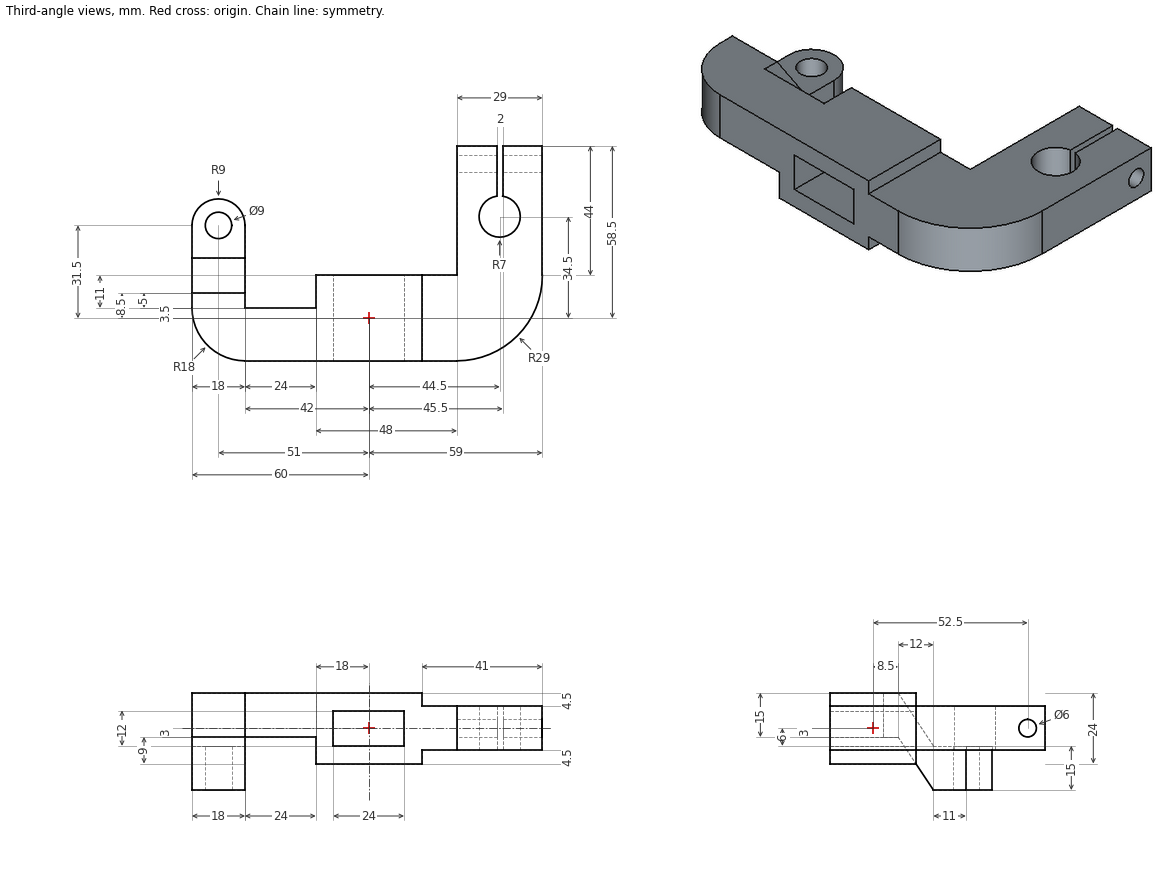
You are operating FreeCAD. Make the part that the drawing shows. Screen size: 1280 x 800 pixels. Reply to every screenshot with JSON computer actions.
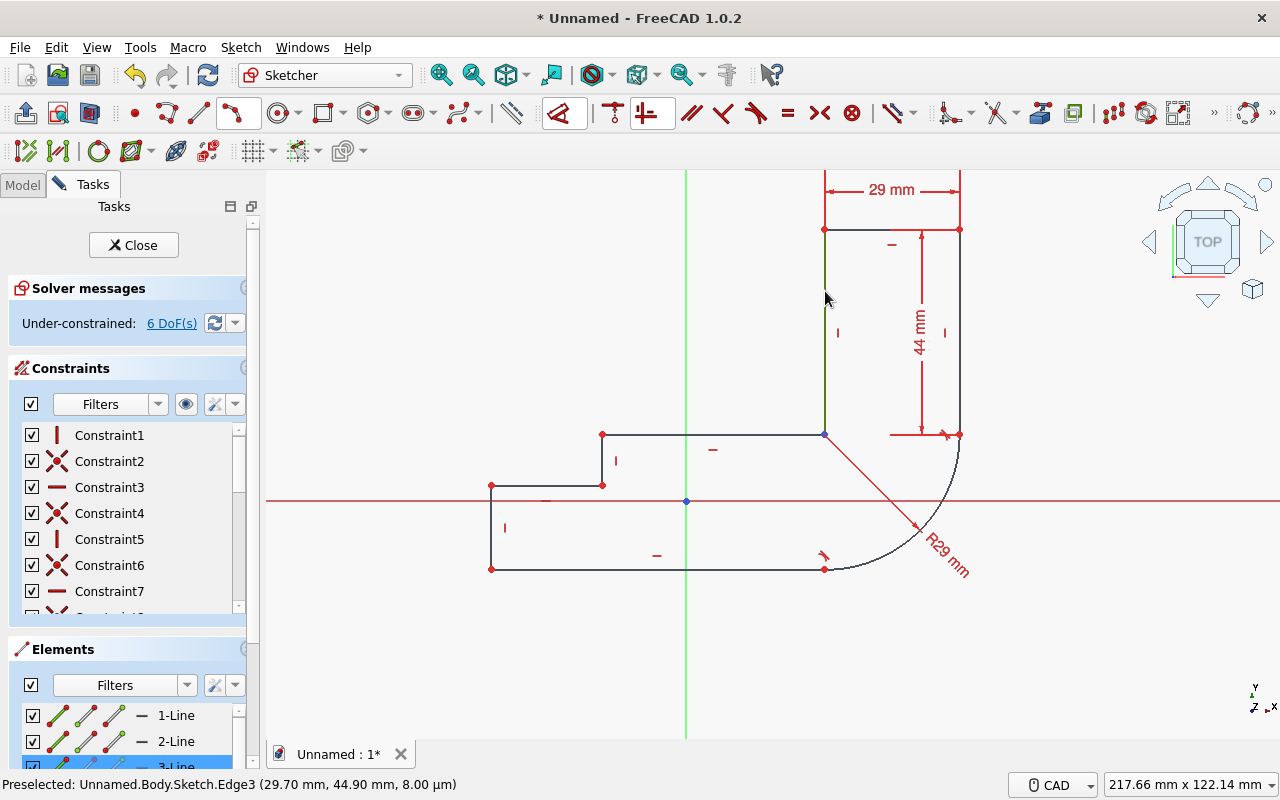
{"action": "key", "text": "i"}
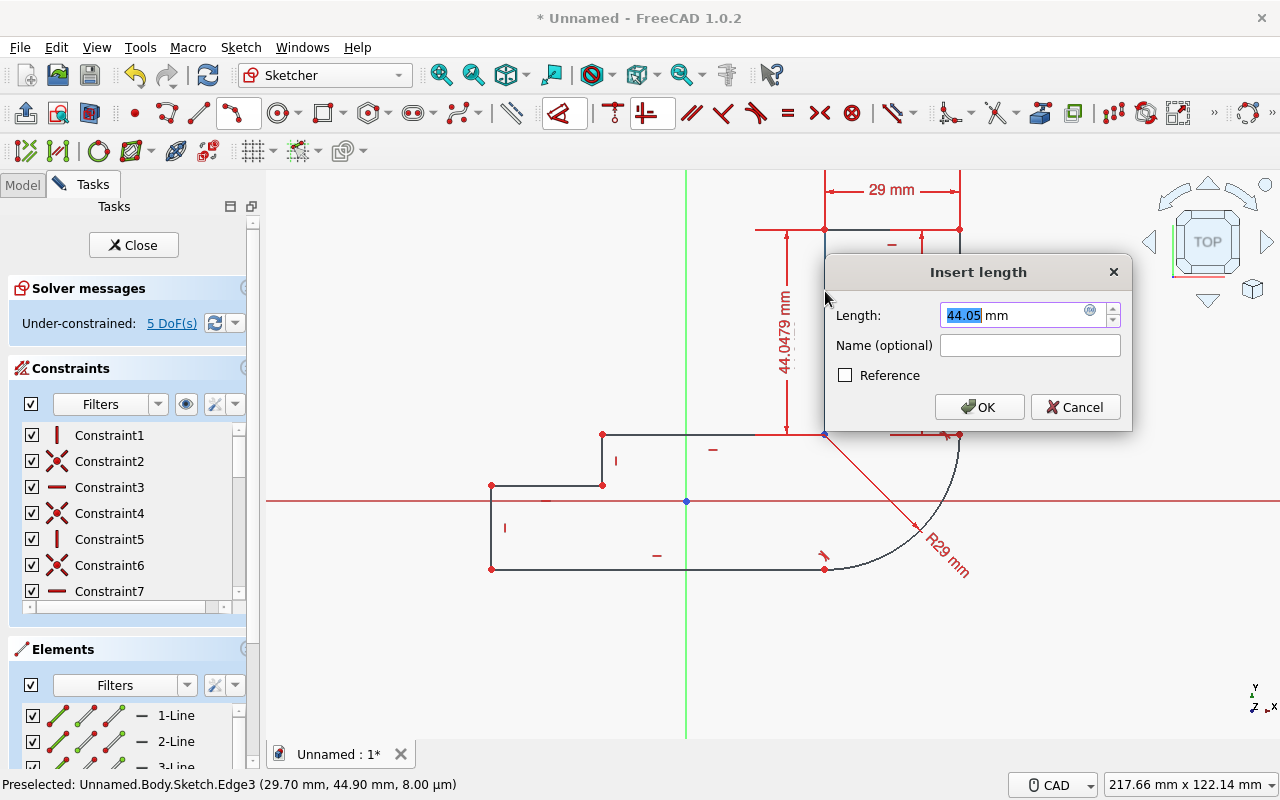
{"action": "type", "text": "44"}
{"action": "key", "text": "Return"}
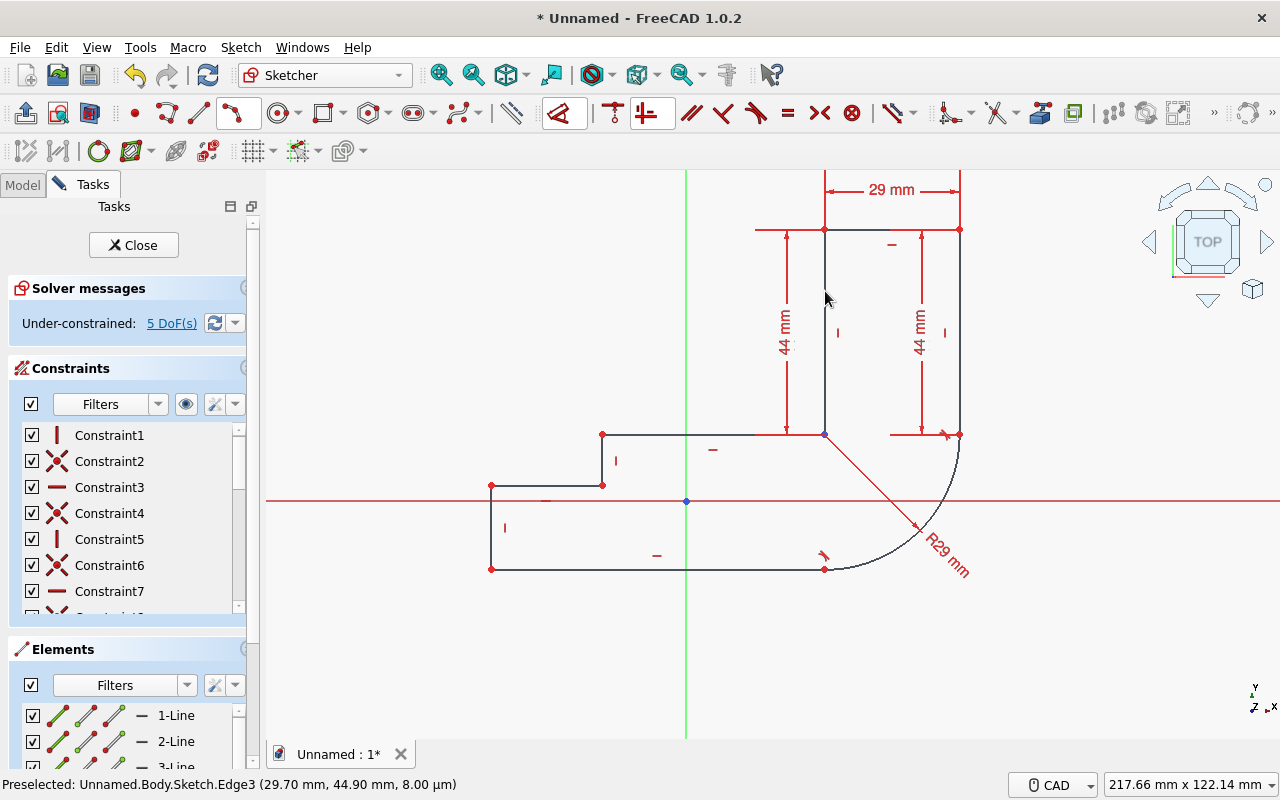
{"action": "left_click", "coordinate": [758, 435]}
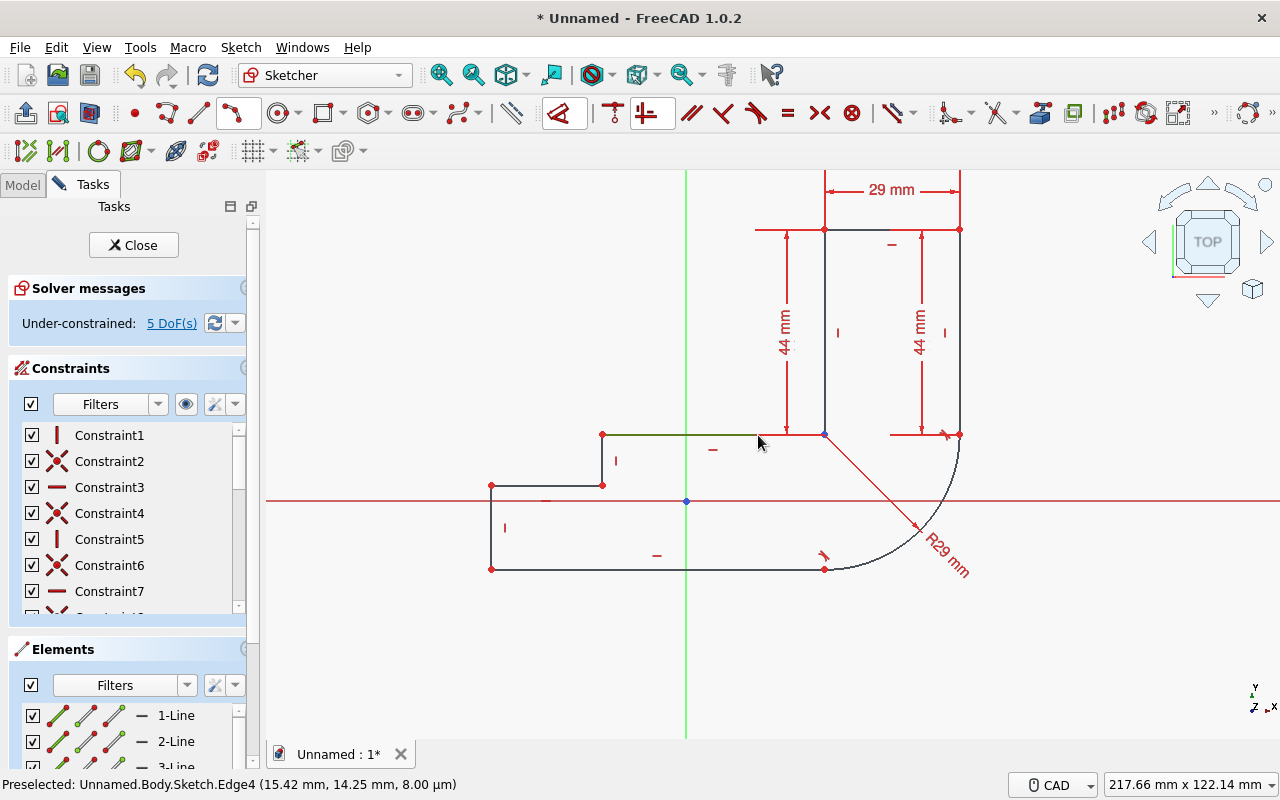
{"action": "key", "text": "l"}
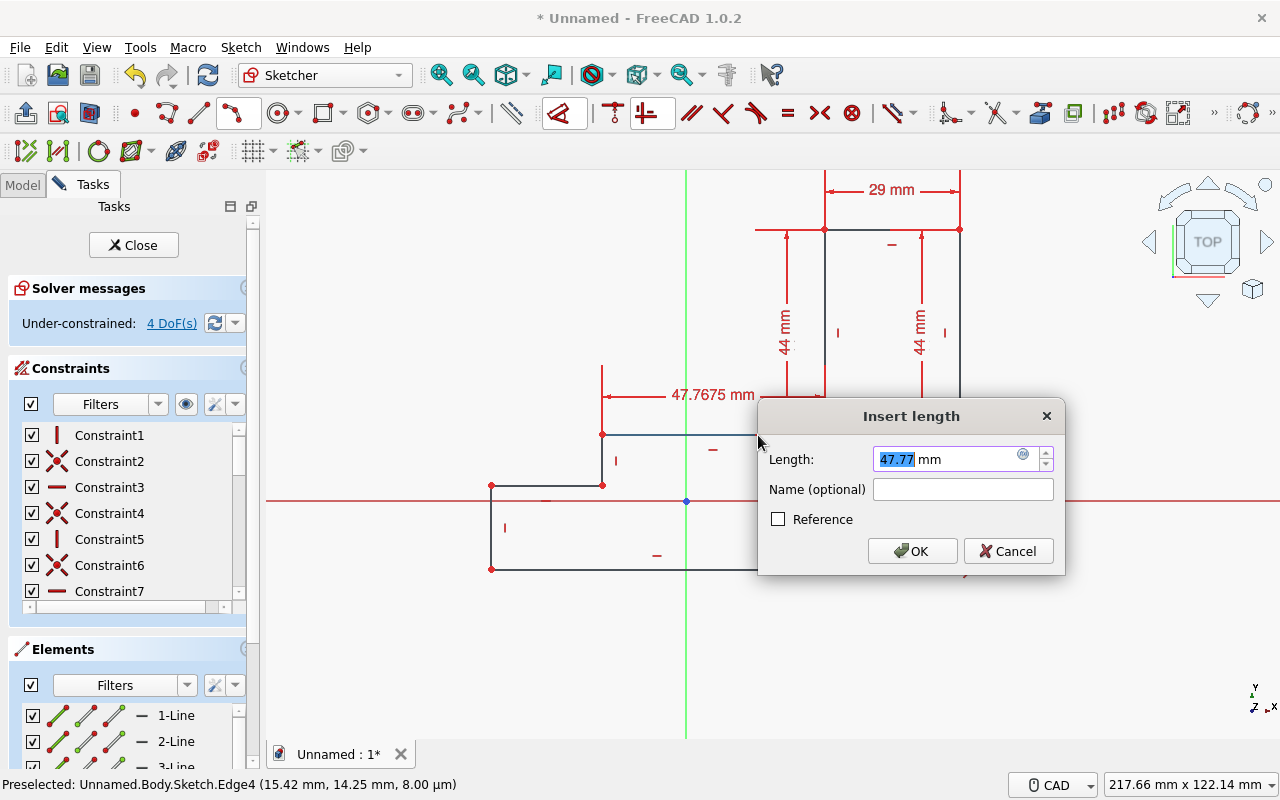
{"action": "type", "text": "48"}
{"action": "key", "text": "Return"}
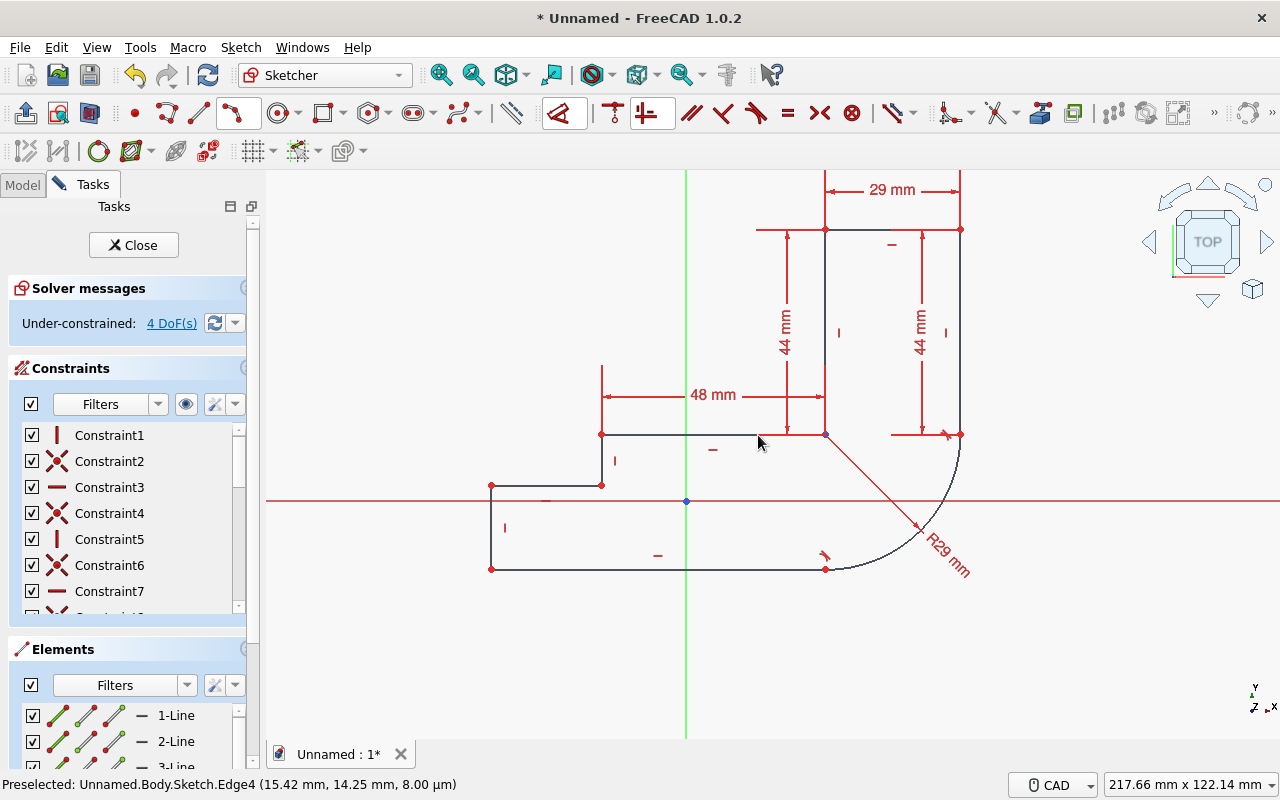
{"action": "left_click", "coordinate": [602, 450]}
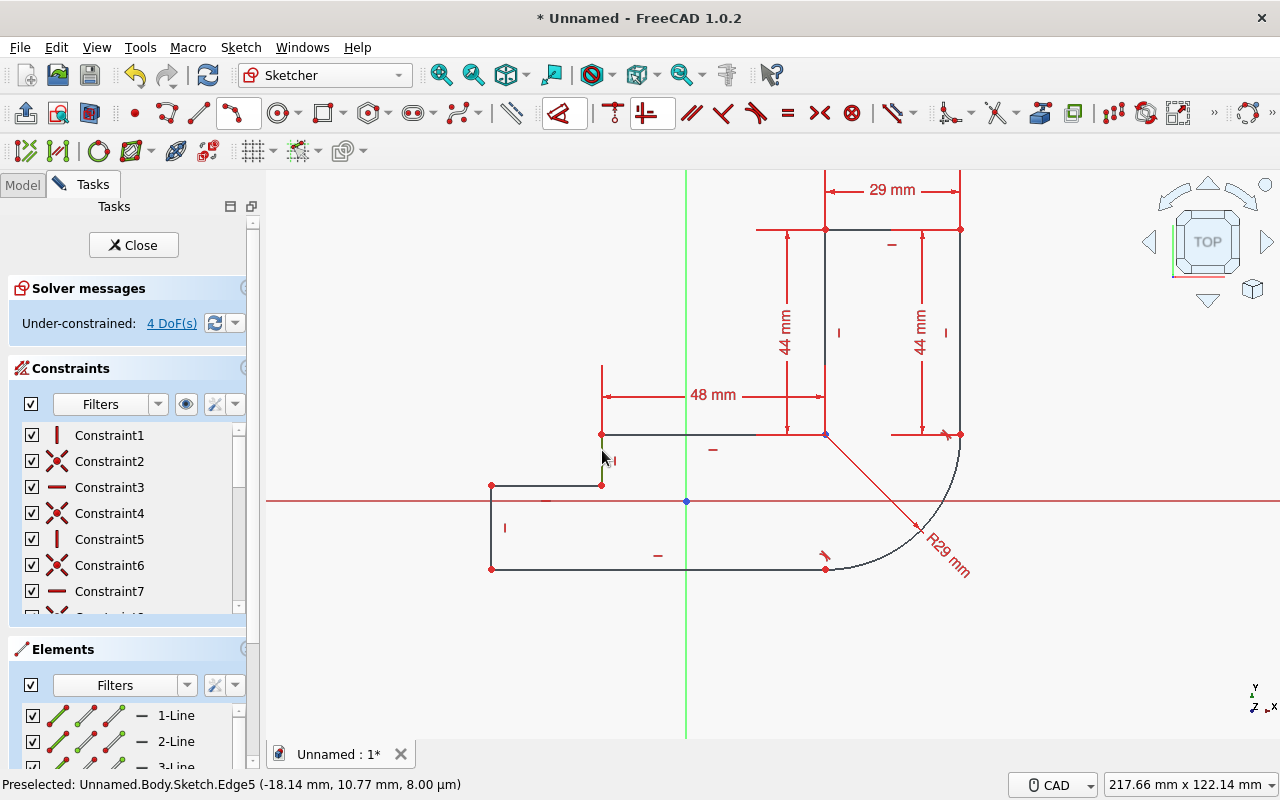
{"action": "left_click", "coordinate": [582, 114]}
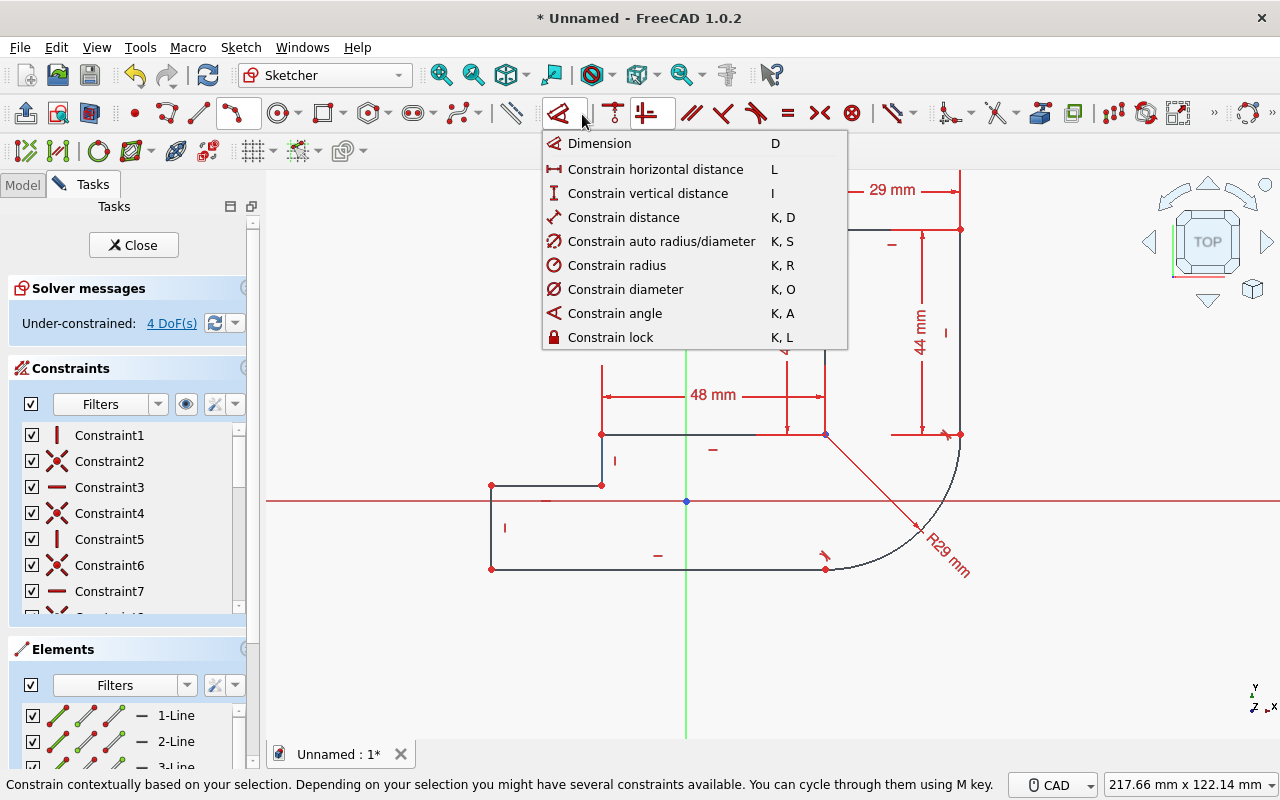
{"action": "left_click", "coordinate": [695, 193]}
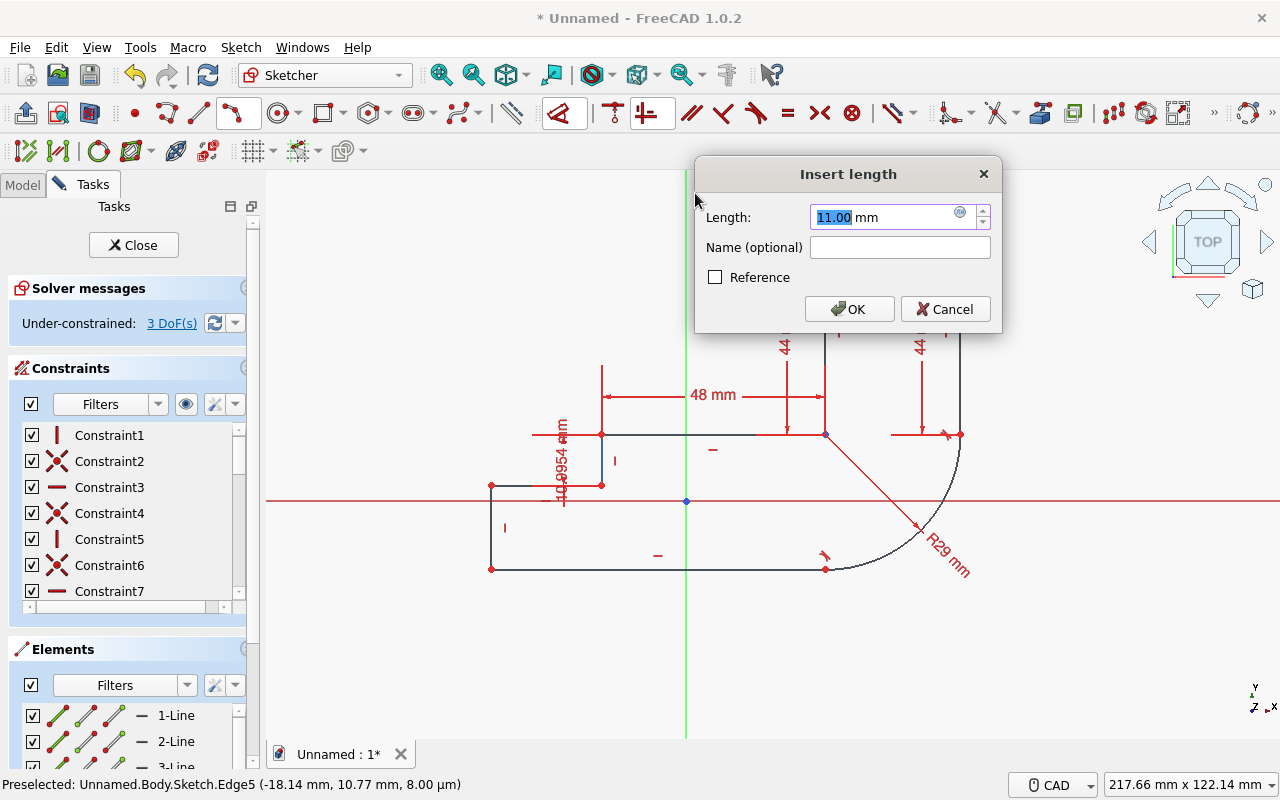
{"action": "type", "text": "11"}
{"action": "key", "text": "Return"}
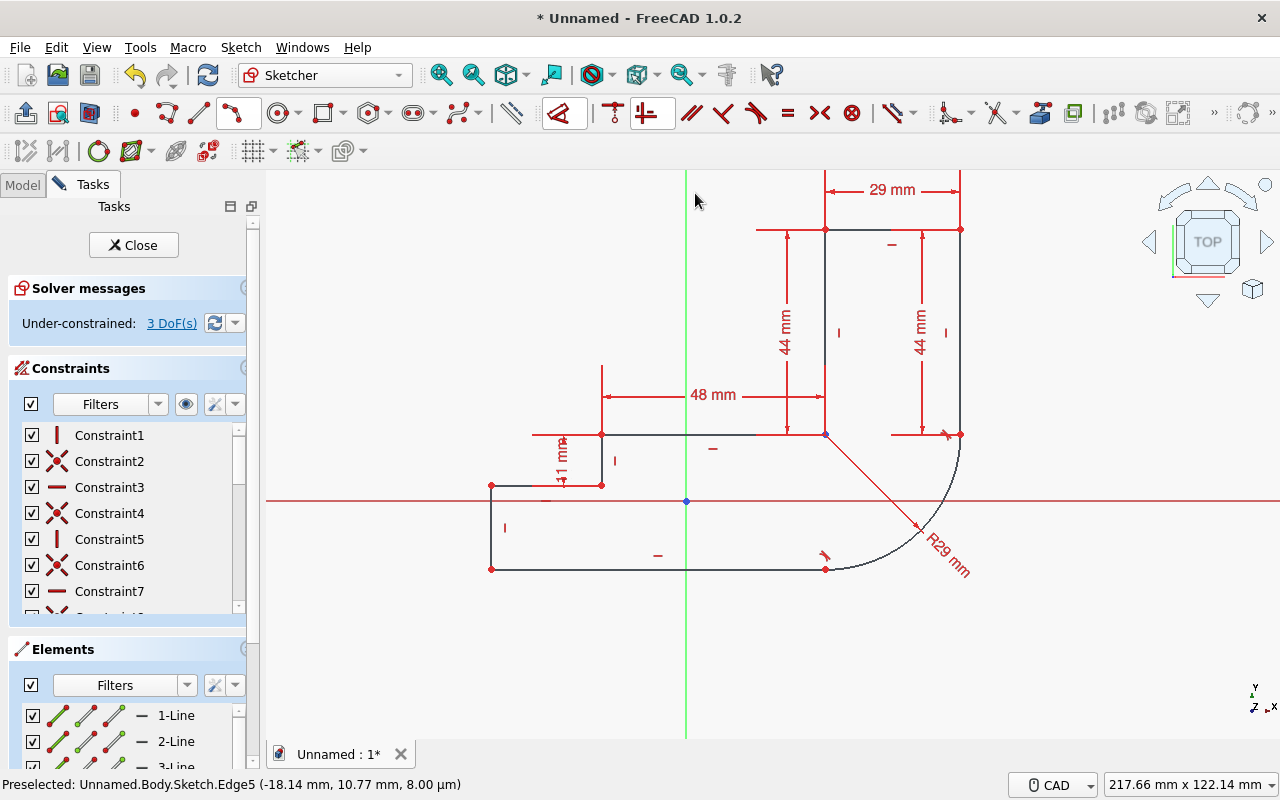
{"action": "left_click", "coordinate": [568, 486]}